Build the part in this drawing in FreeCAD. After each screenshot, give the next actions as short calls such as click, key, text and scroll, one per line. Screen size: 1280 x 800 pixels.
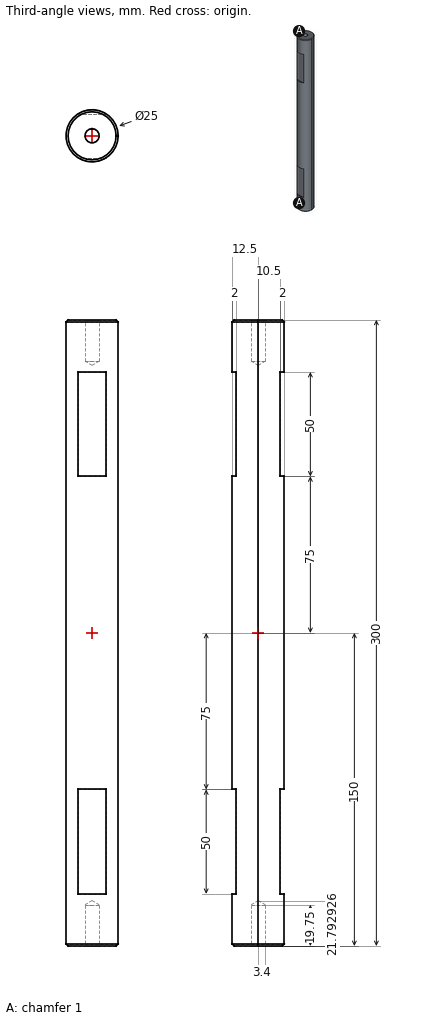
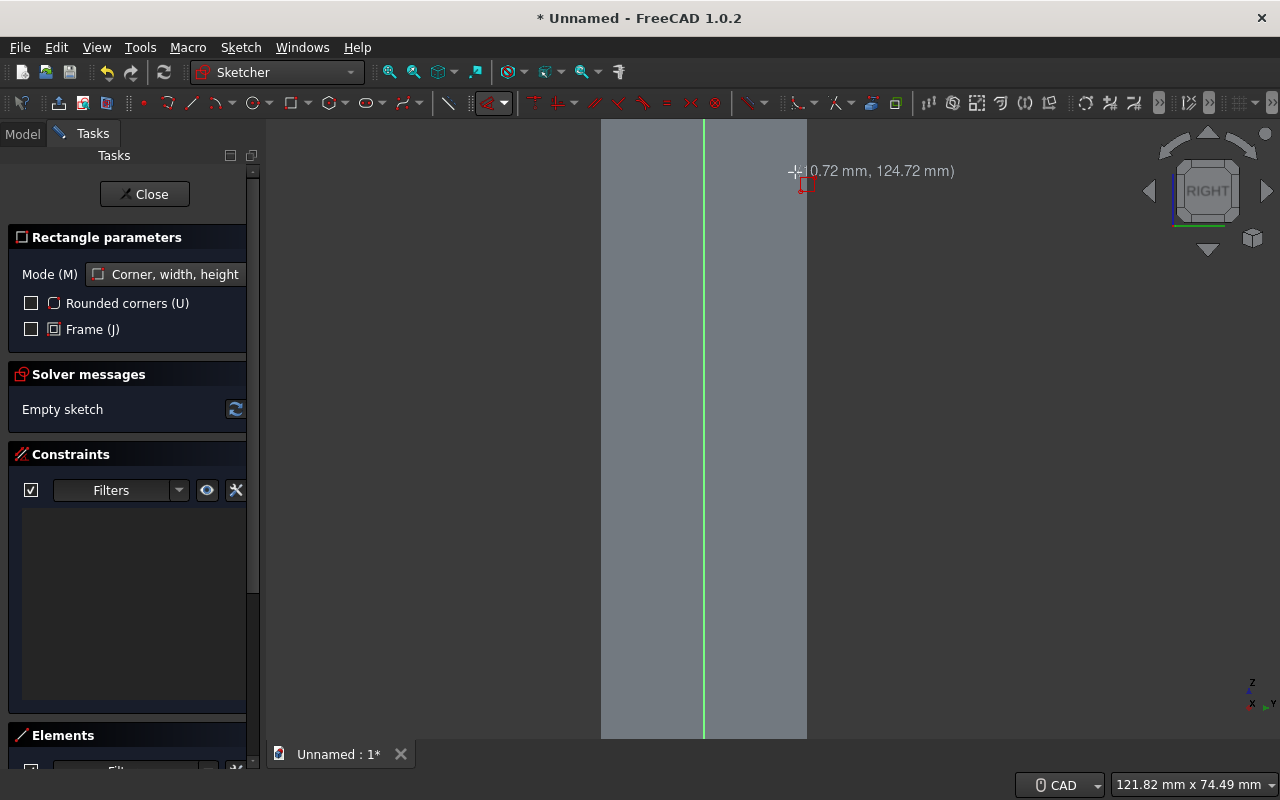
scroll(705, 230, down, 8)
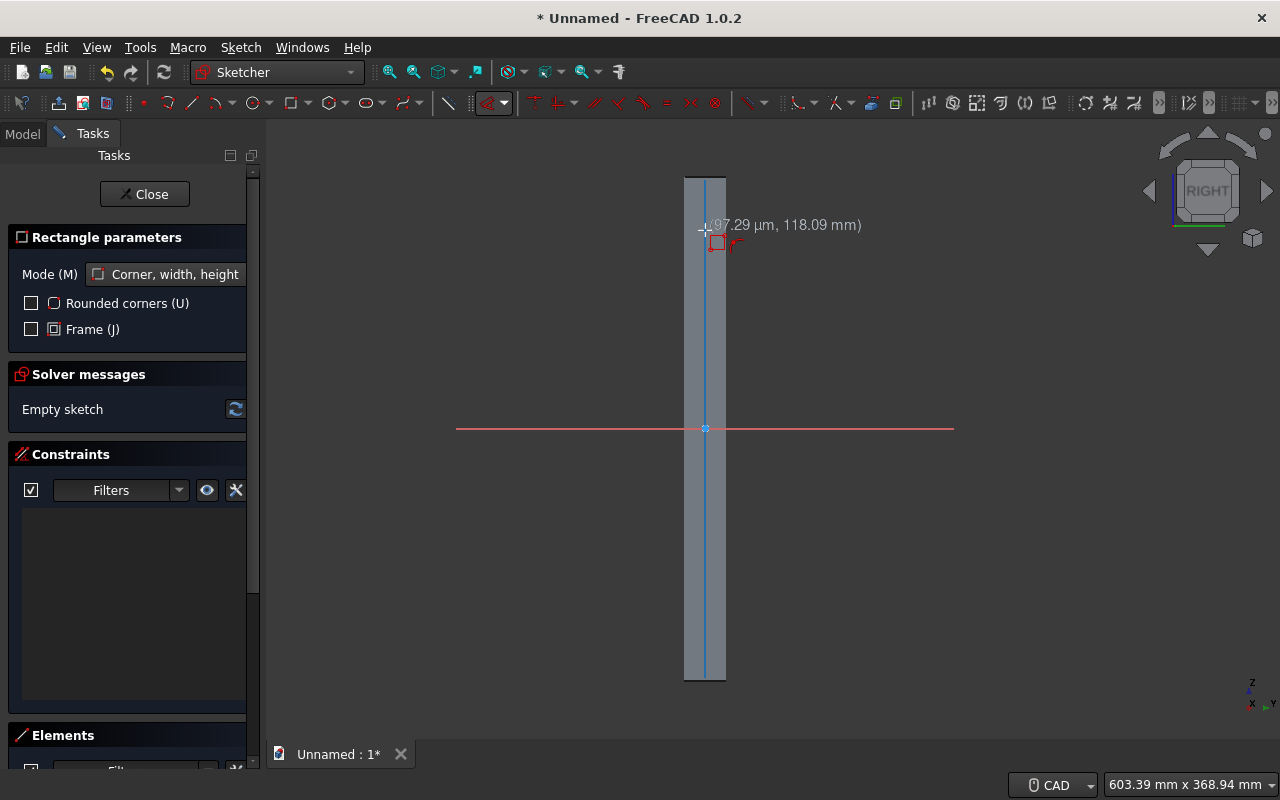
click(723, 219)
move(726, 303)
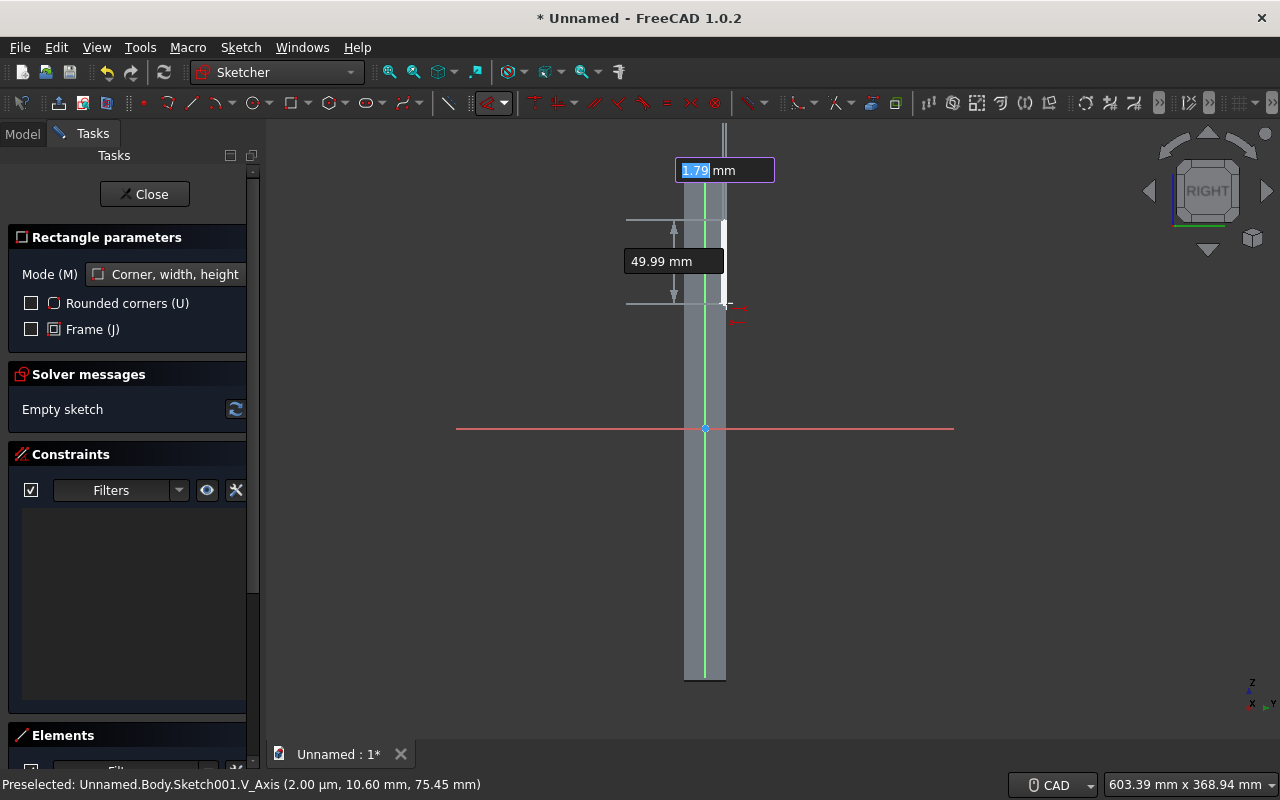
text(2)
key(Tab)
text(50)
key(Return)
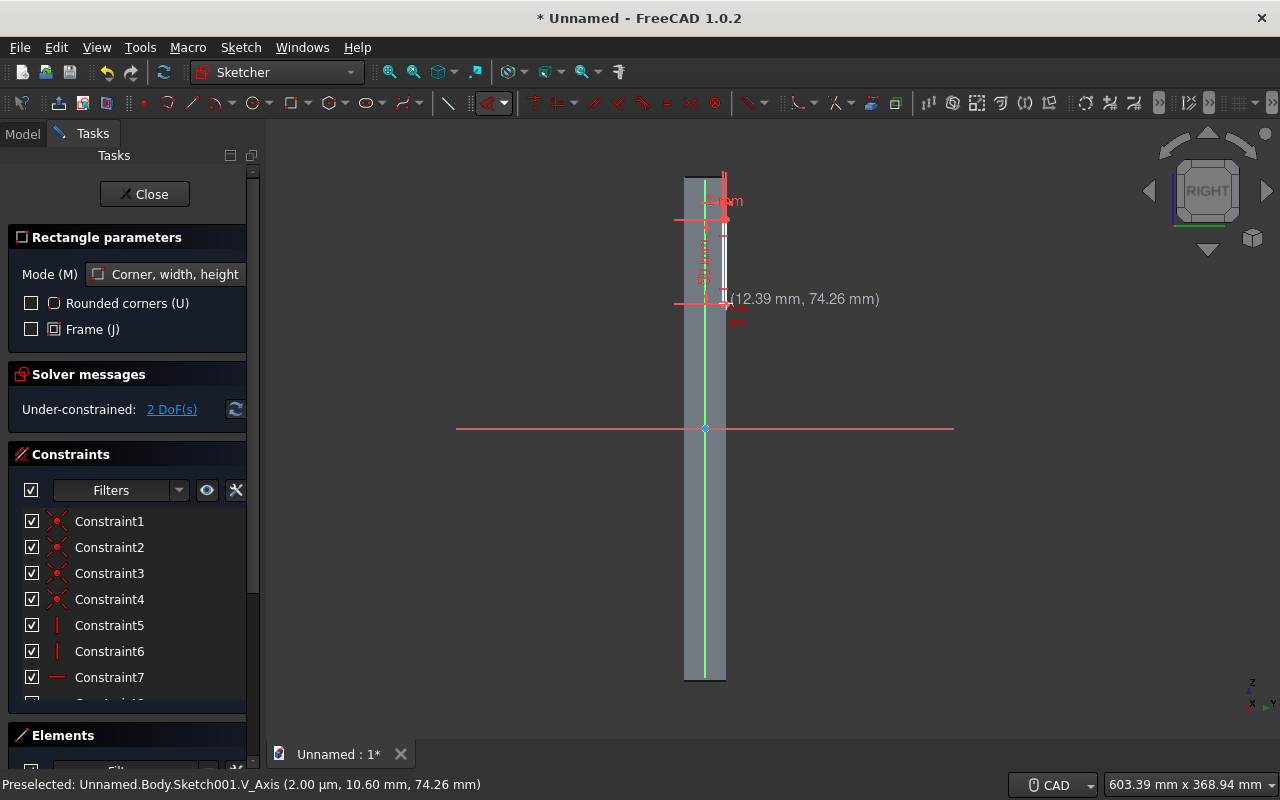
scroll(684, 219, up, 8)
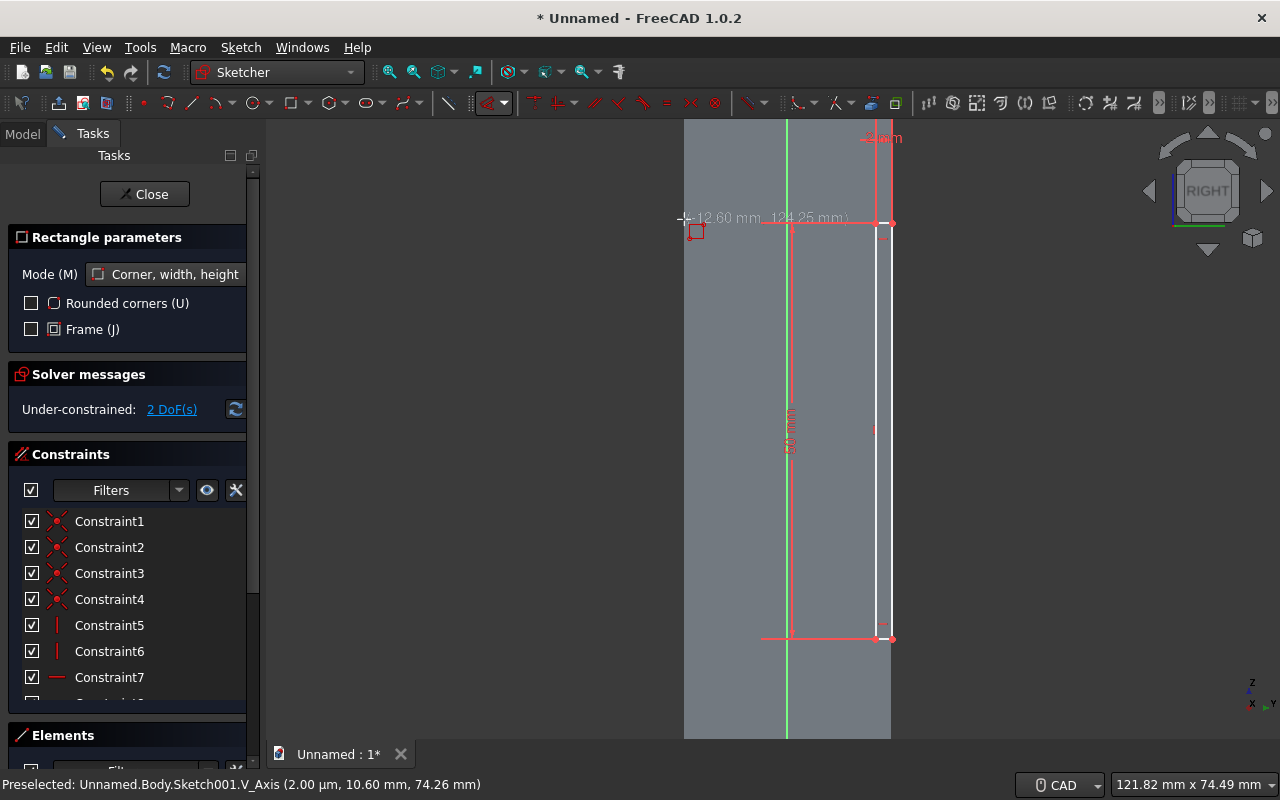
scroll(684, 219, down, 8)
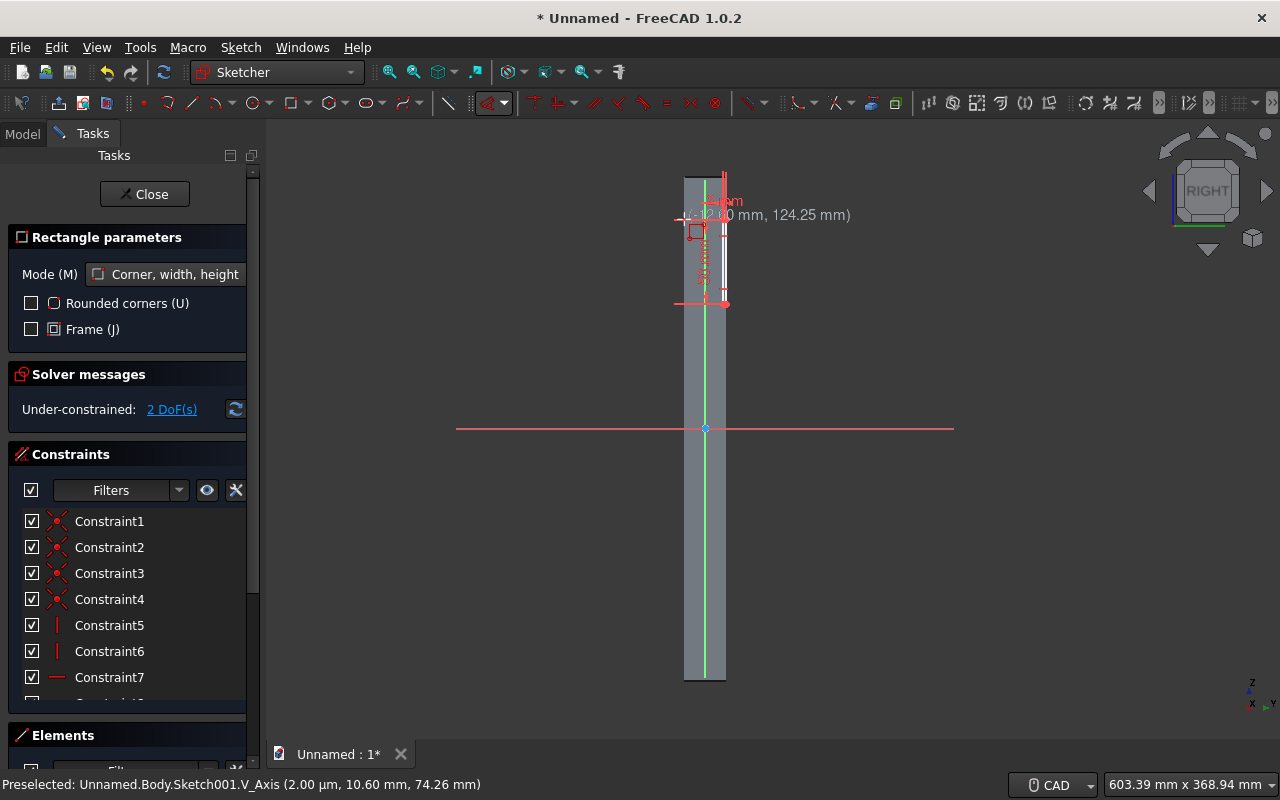
click(684, 219)
move(688, 303)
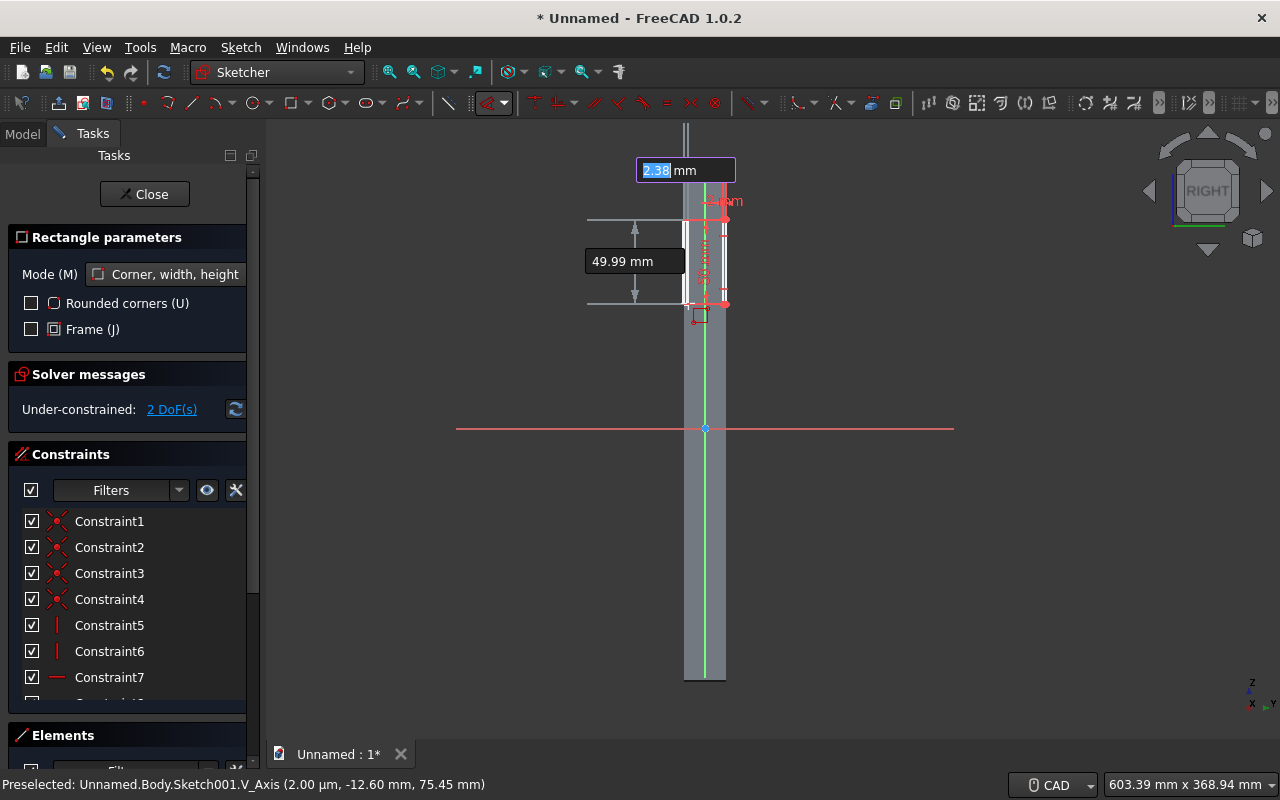
text(2)
key(Tab)
text(50)
key(Return)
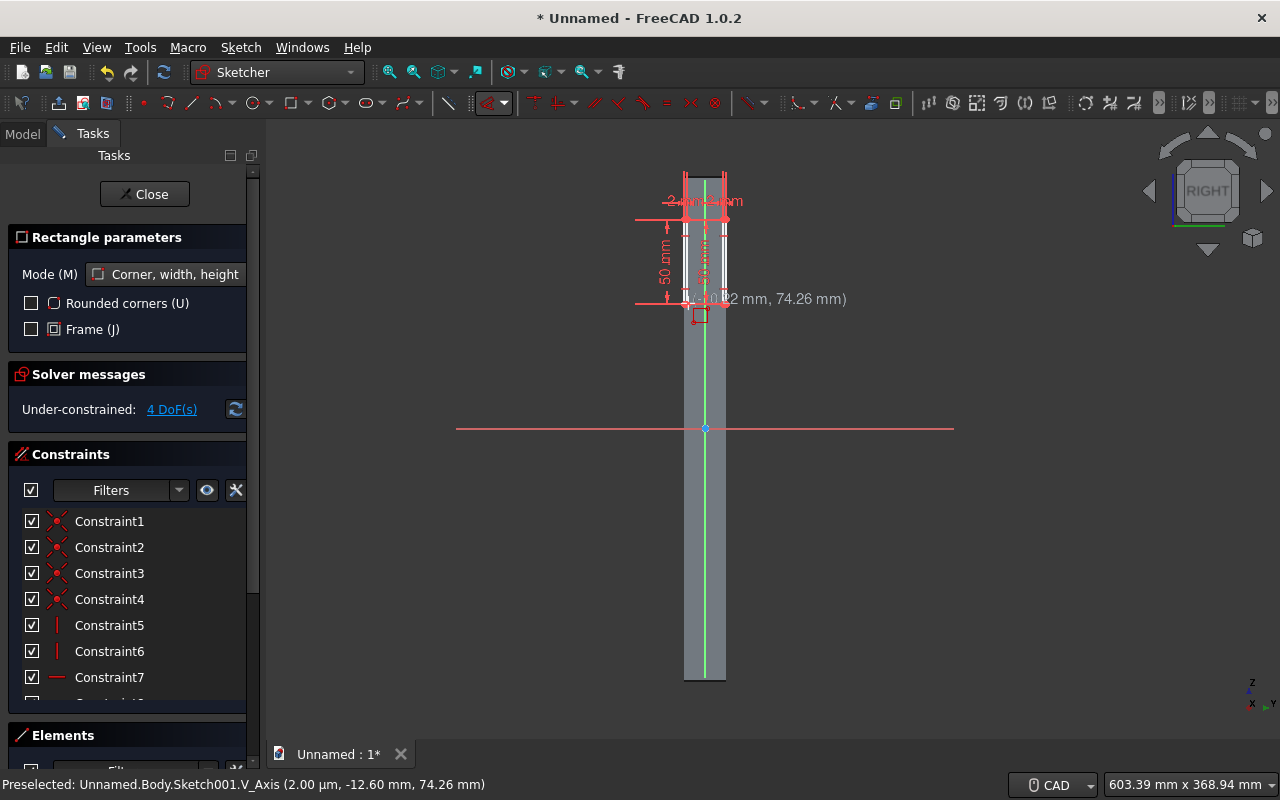
scroll(684, 555, up, 8)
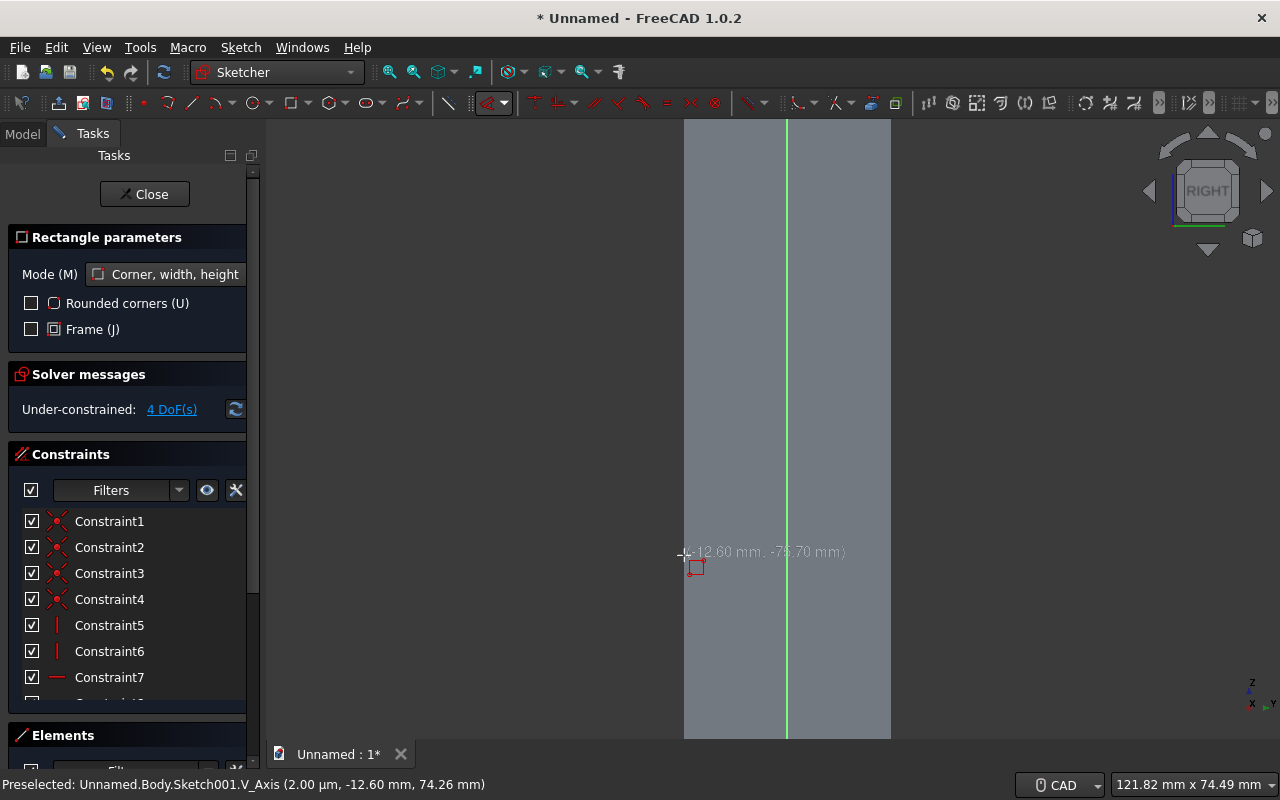
scroll(684, 556, down, 8)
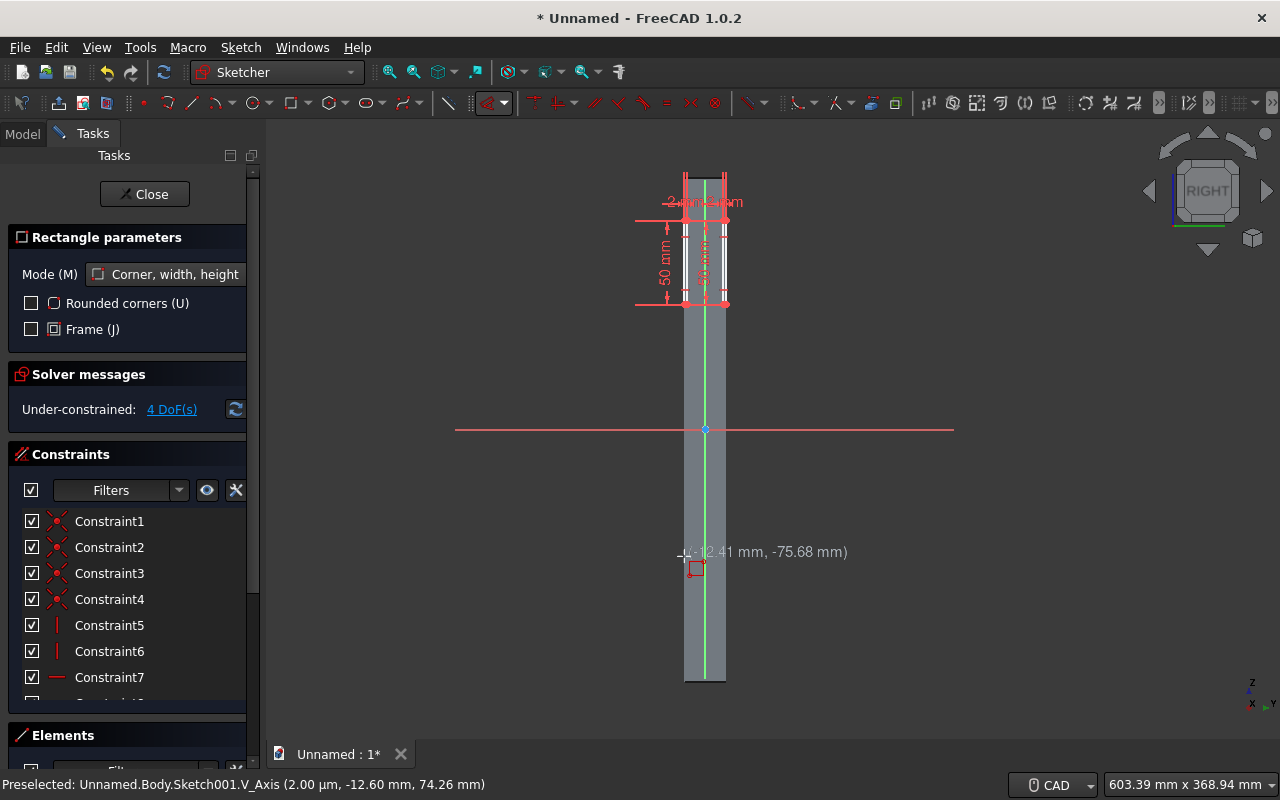
click(684, 556)
move(688, 640)